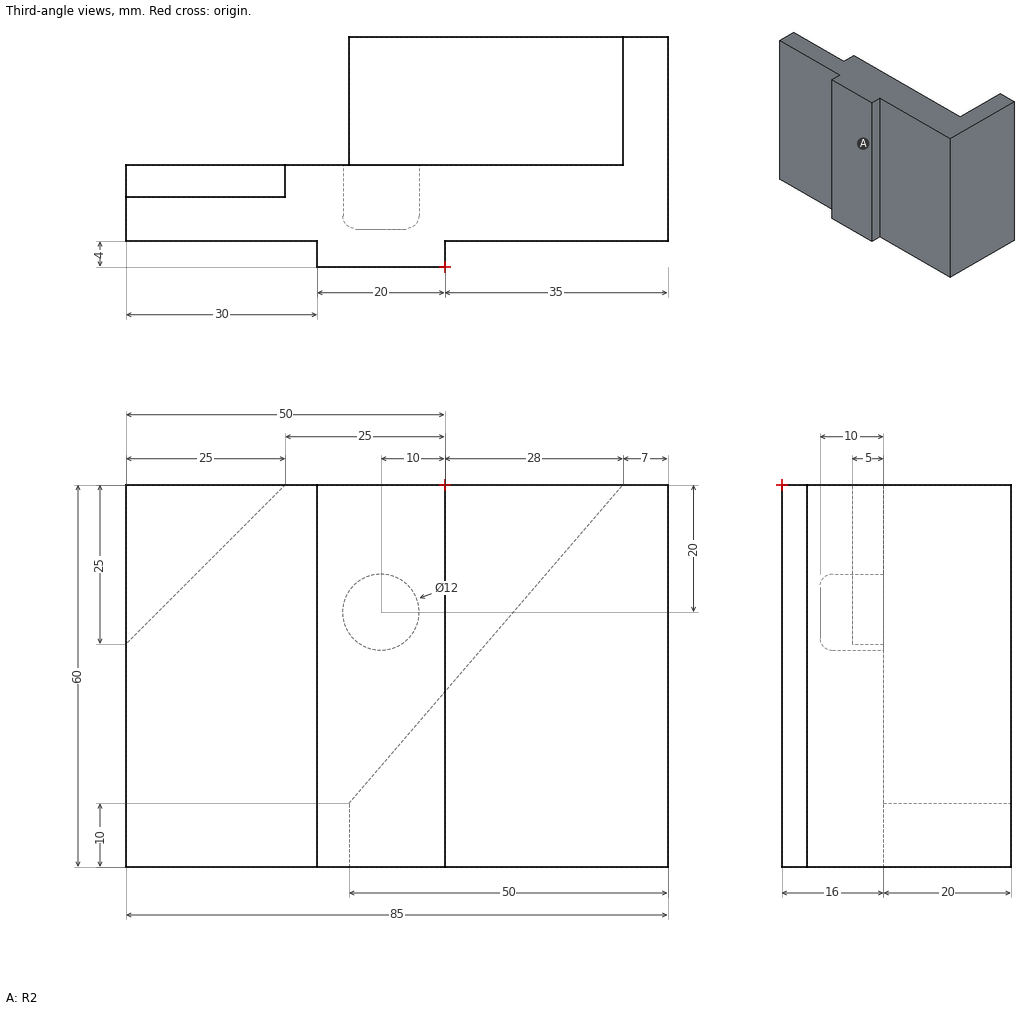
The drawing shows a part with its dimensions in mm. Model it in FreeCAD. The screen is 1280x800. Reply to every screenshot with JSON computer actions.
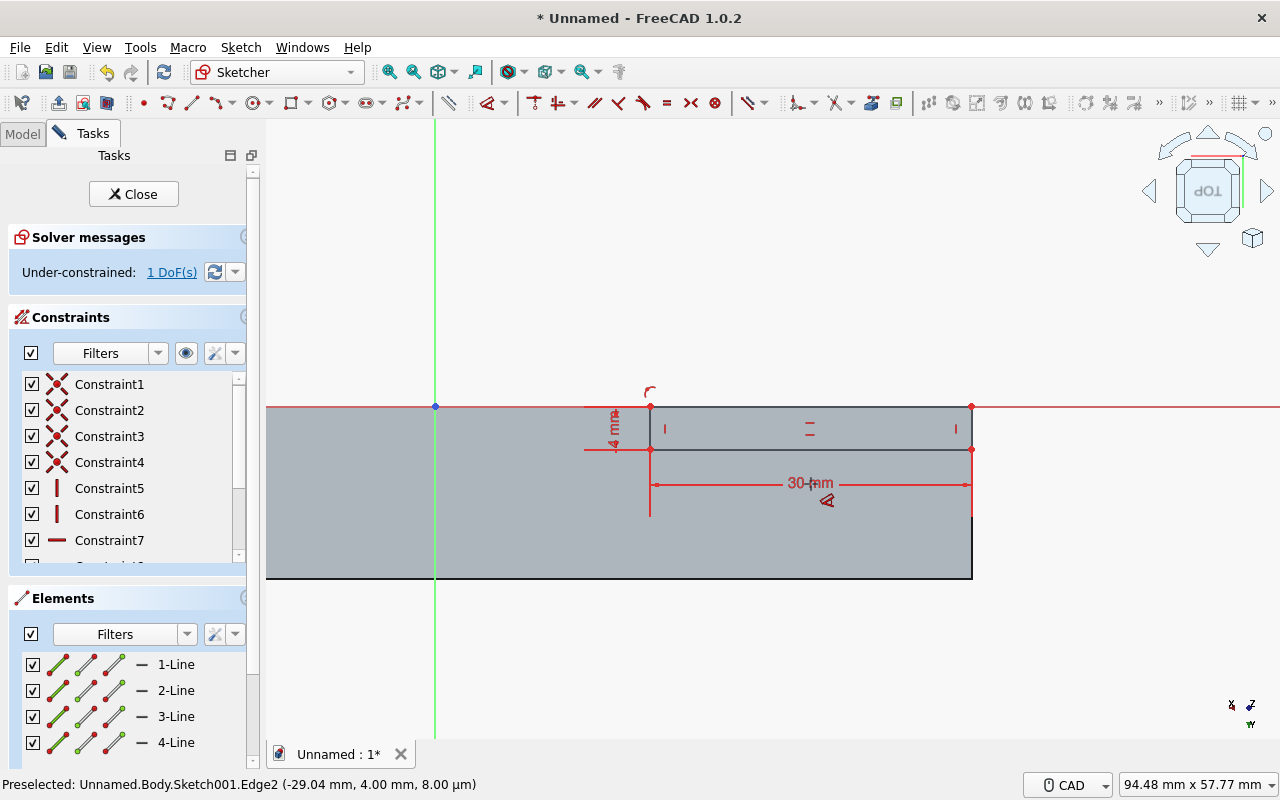
{"action": "left_click", "coordinate": [650, 407]}
{"action": "left_click", "coordinate": [543, 373]}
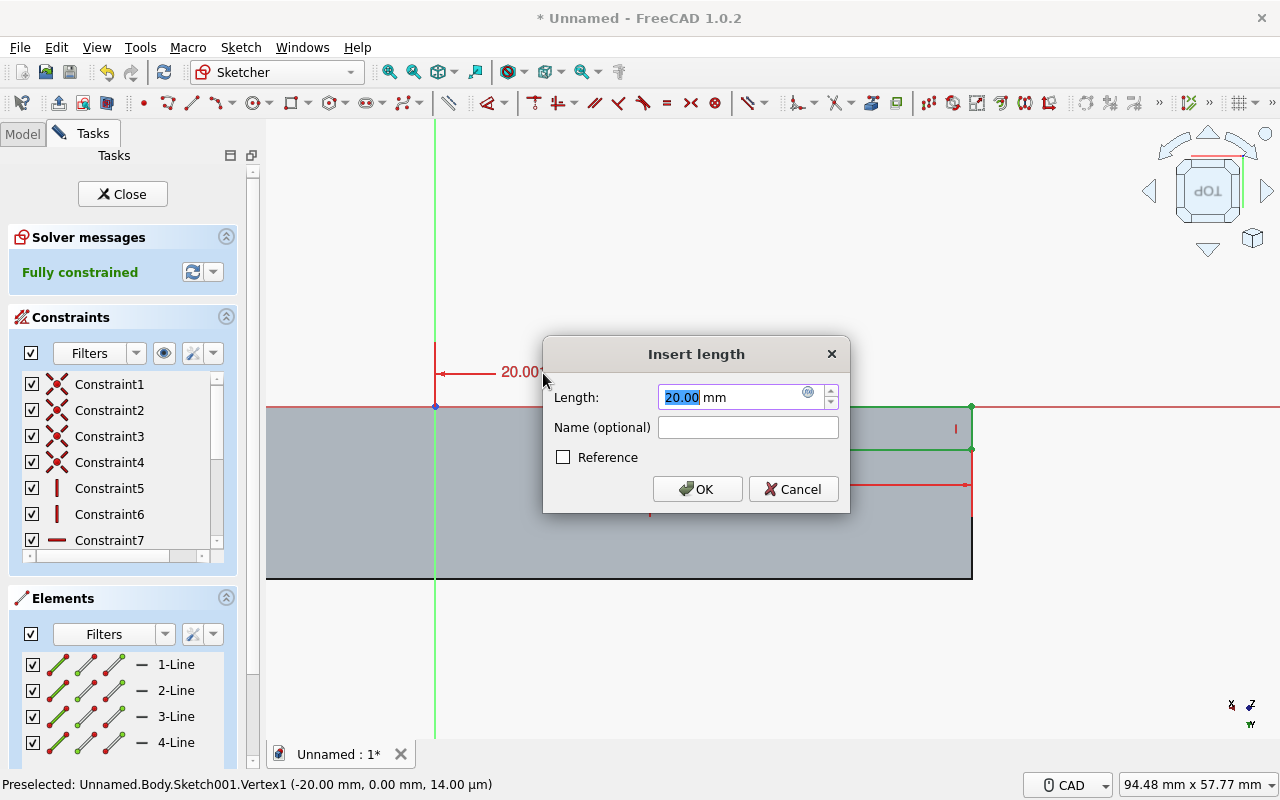
{"action": "type", "text": "20"}
{"action": "key", "text": "Return"}
{"action": "key", "text": "Escape"}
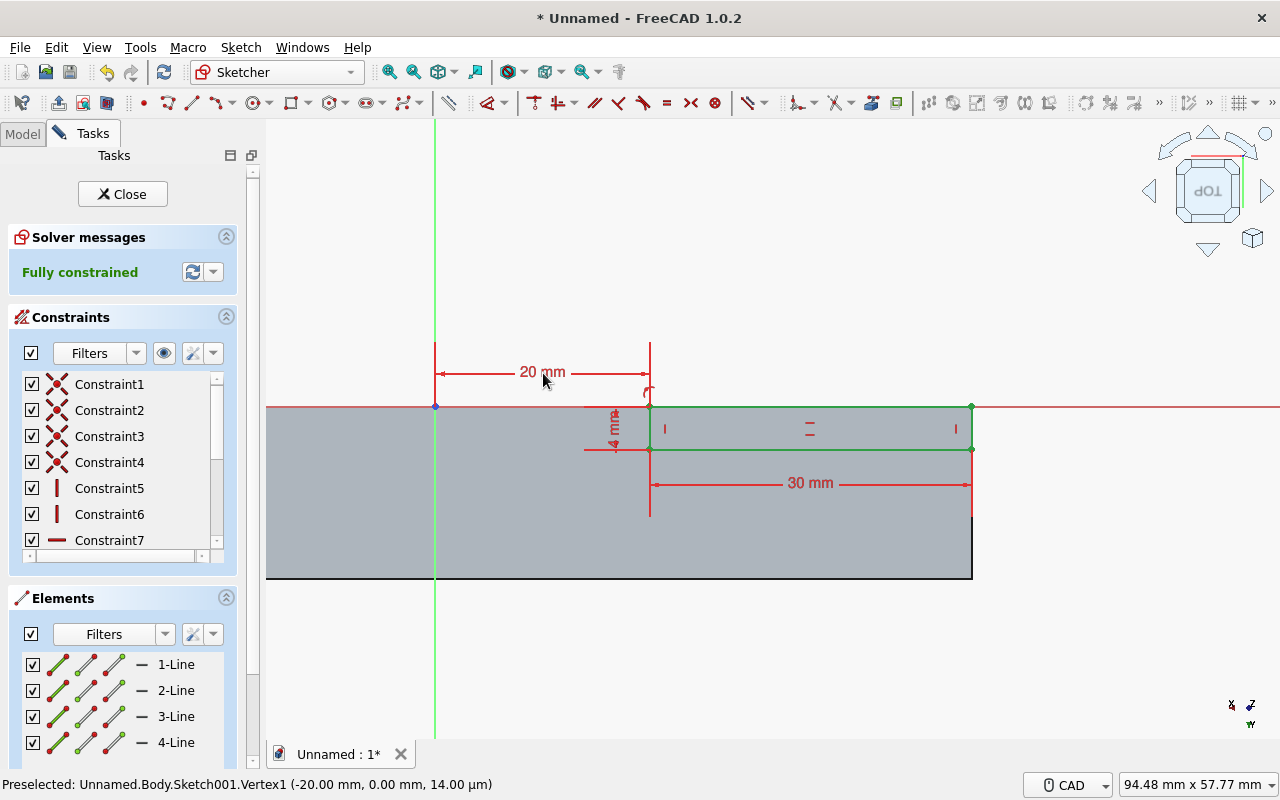
{"action": "left_click", "coordinate": [123, 194]}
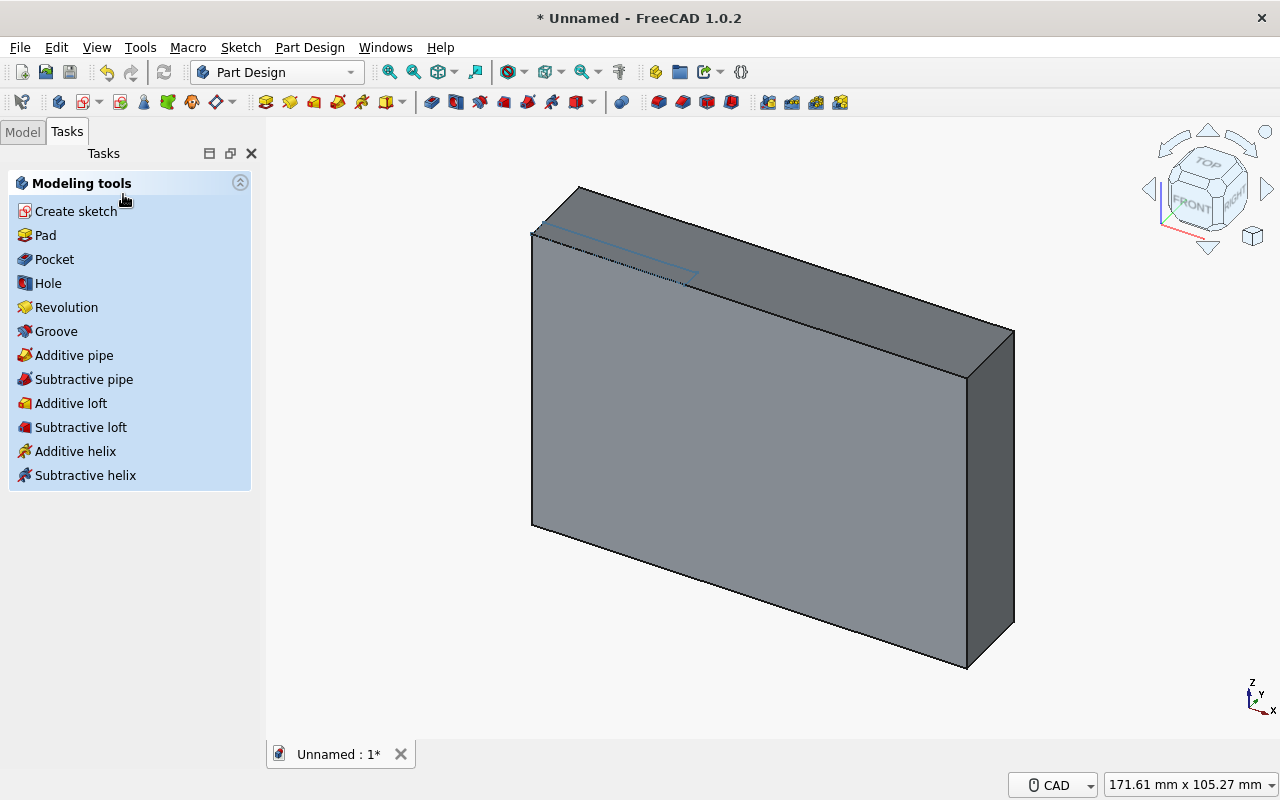
{"action": "left_click", "coordinate": [432, 102]}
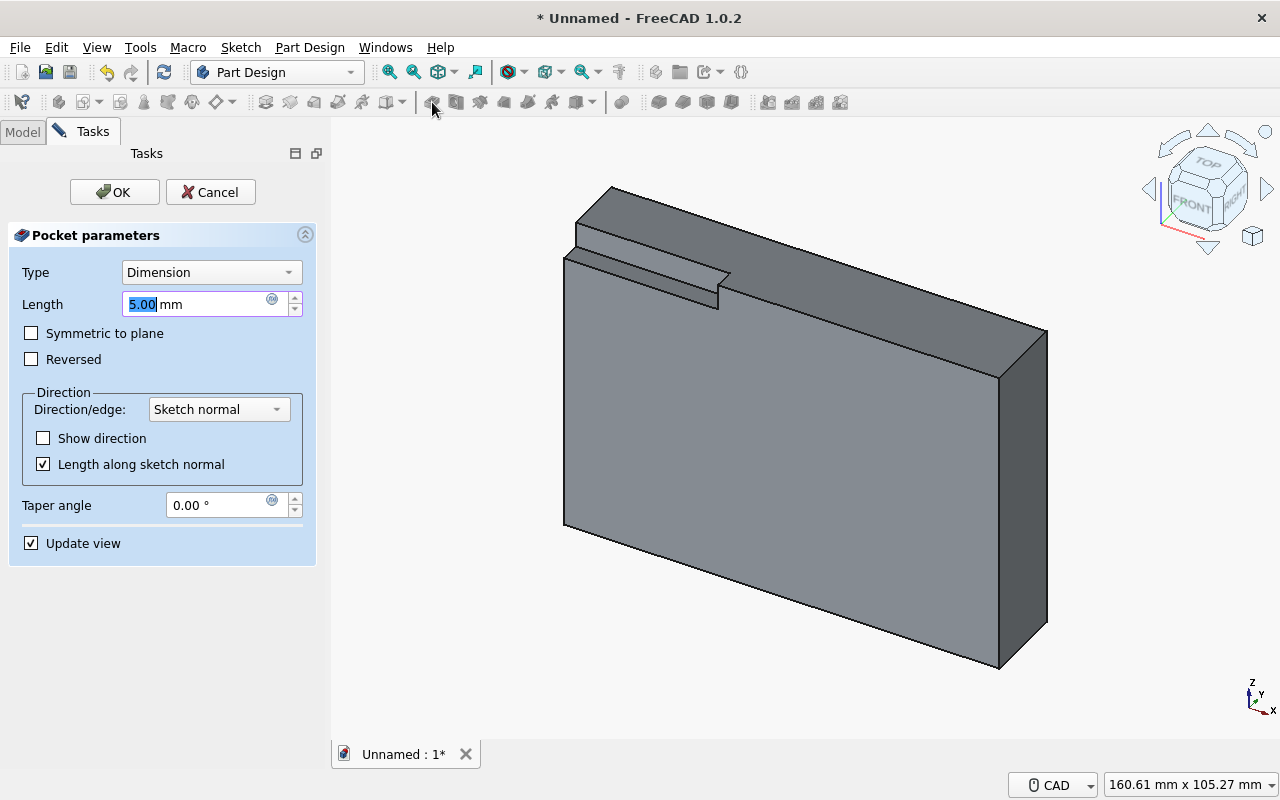
{"action": "left_click", "coordinate": [212, 272]}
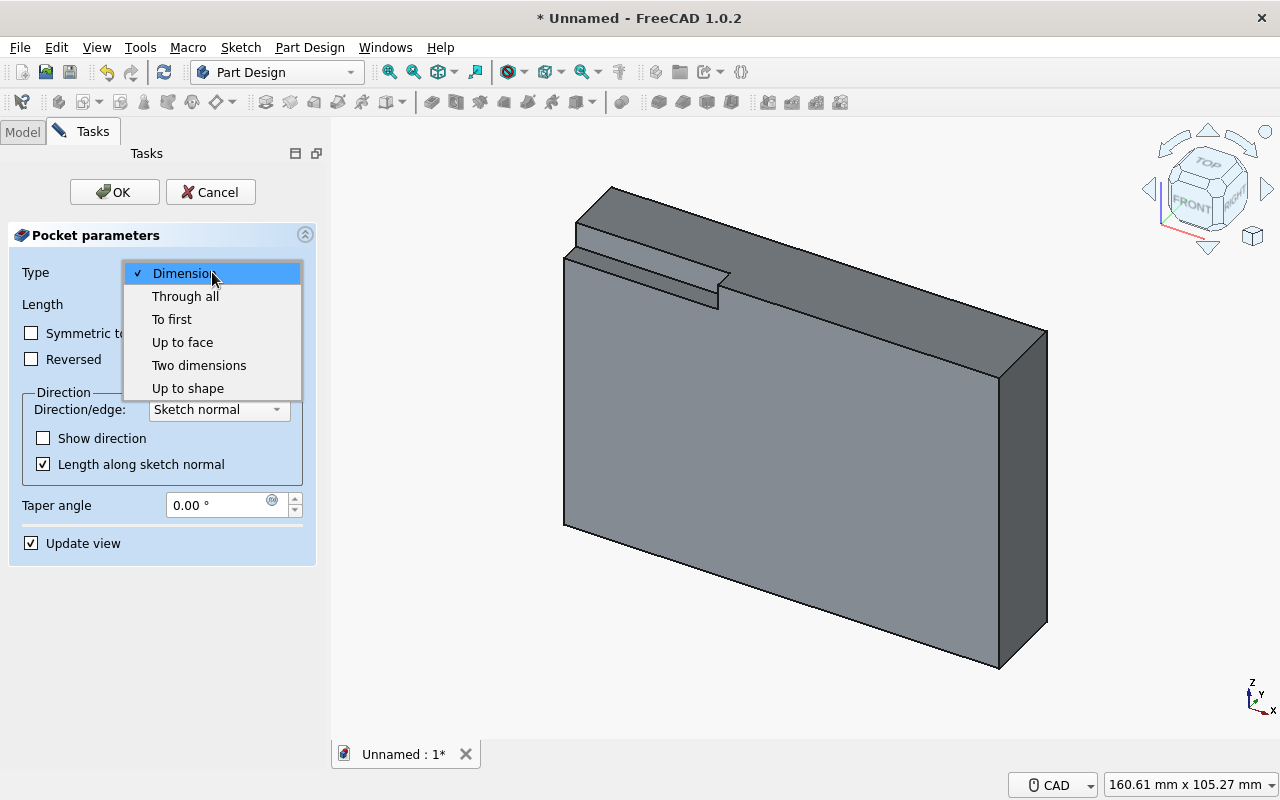
{"action": "left_click", "coordinate": [212, 296]}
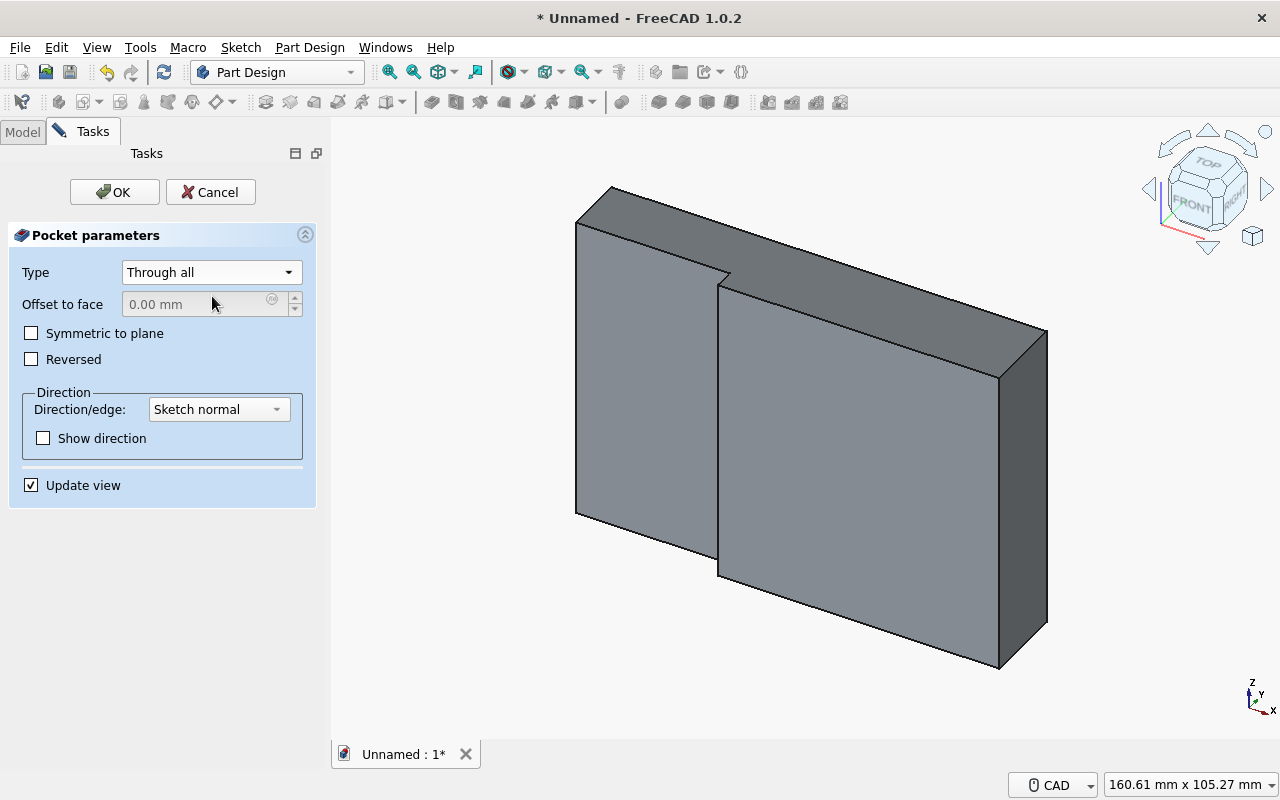
{"action": "left_click", "coordinate": [115, 192]}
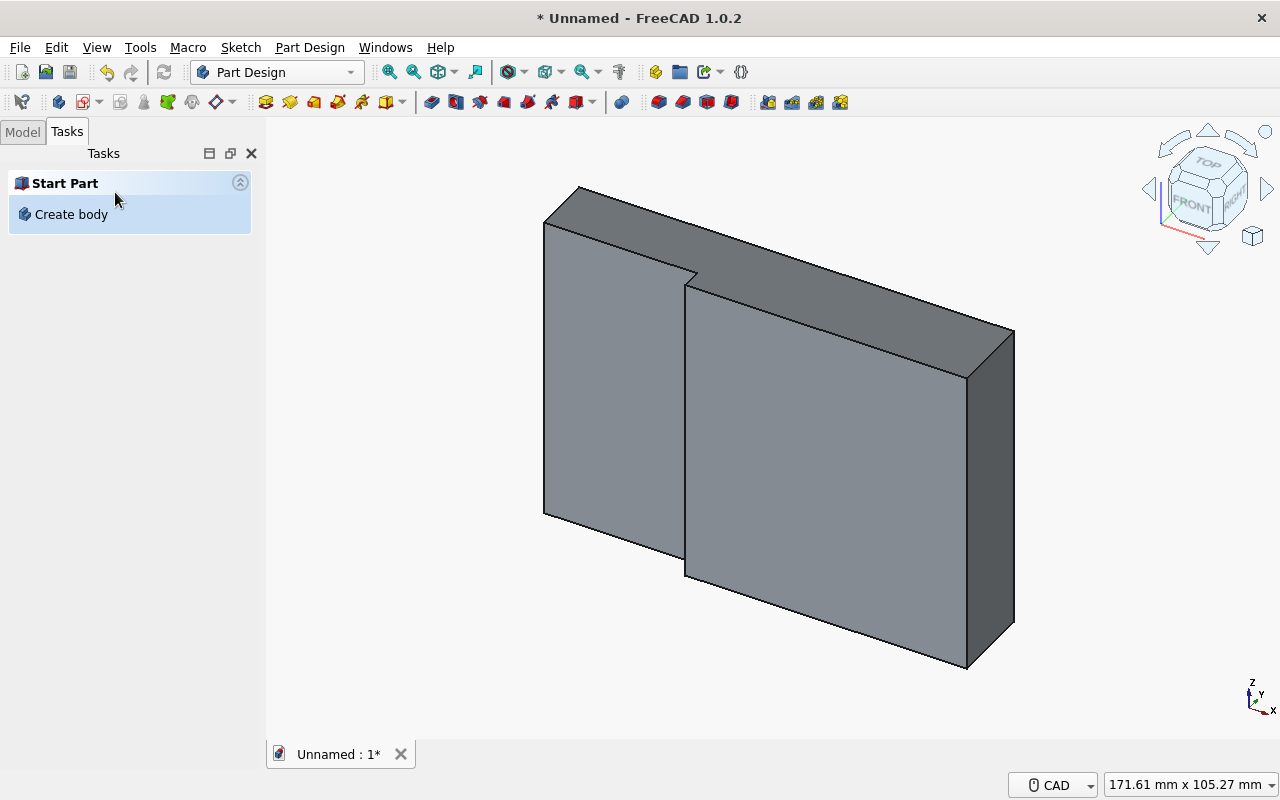
{"action": "left_click", "coordinate": [897, 323]}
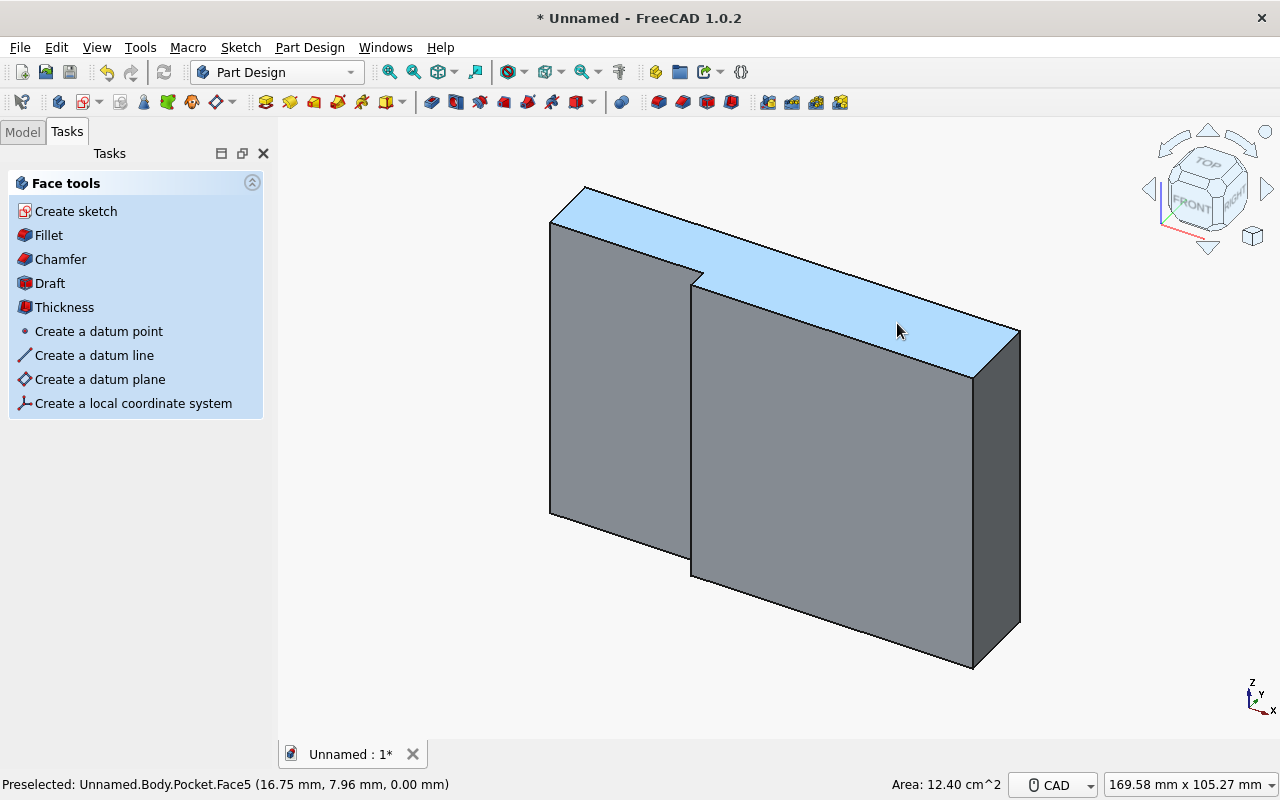
{"action": "left_click", "coordinate": [84, 102]}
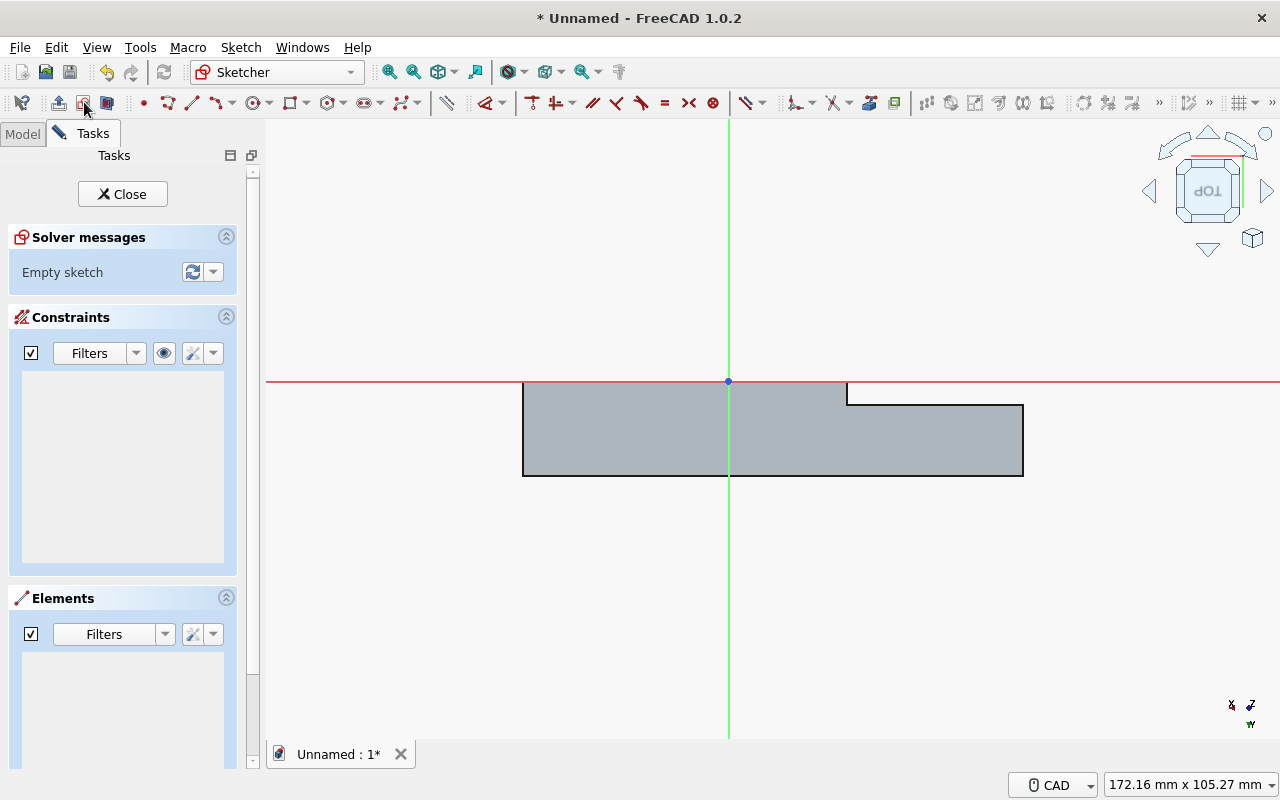
{"action": "scroll", "coordinate": [580, 373], "scroll_direction": "up", "scroll_amount": 5}